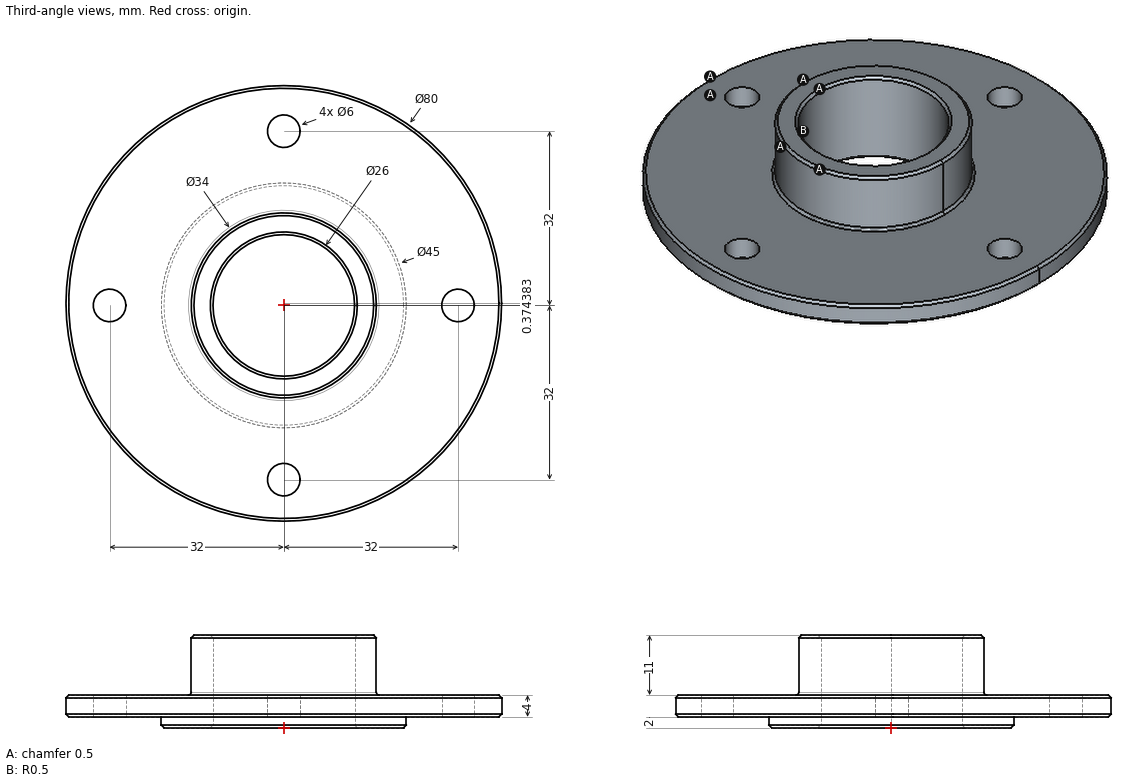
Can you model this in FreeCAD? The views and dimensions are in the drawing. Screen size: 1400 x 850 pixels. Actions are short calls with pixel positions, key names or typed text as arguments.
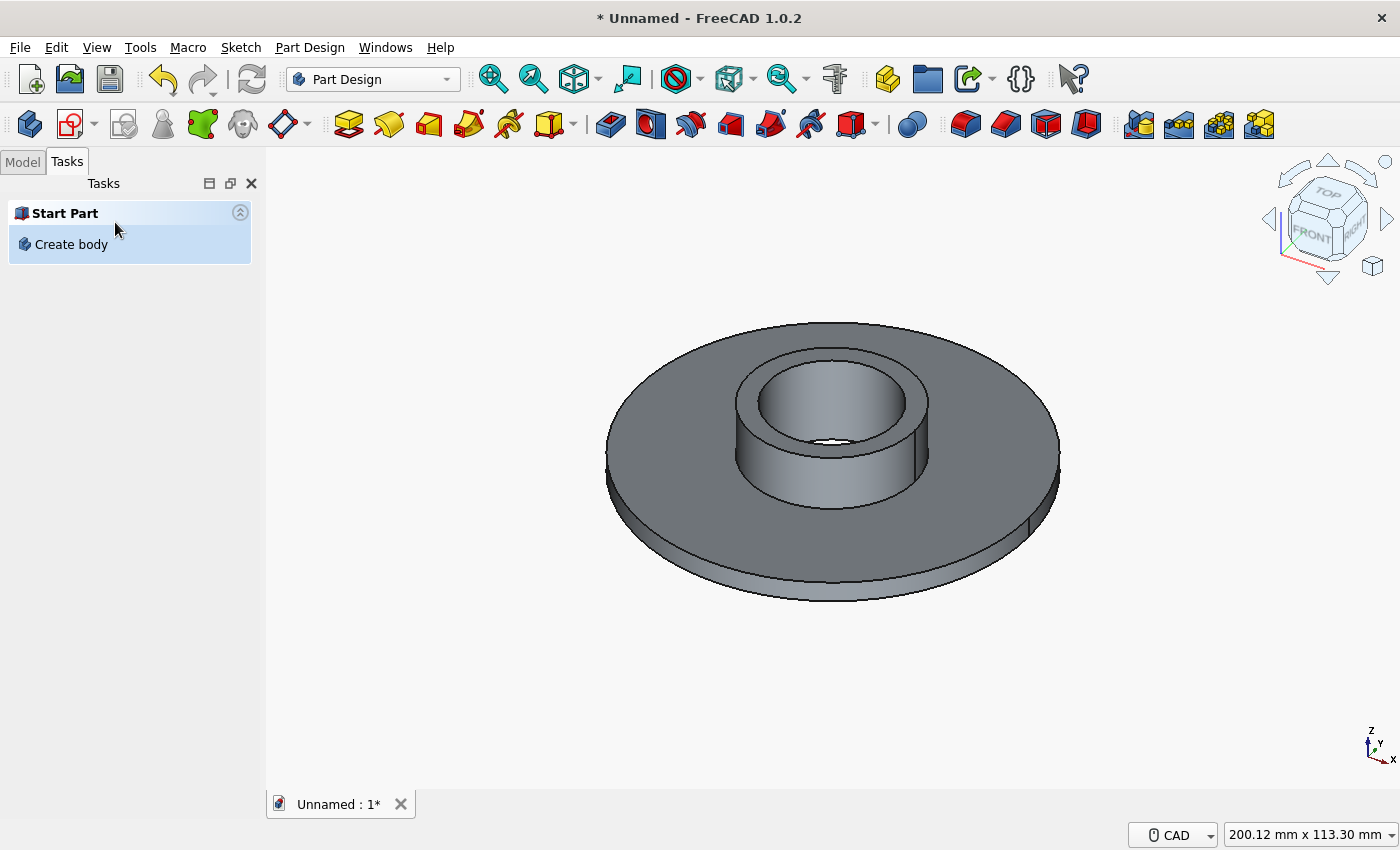
click(736, 407)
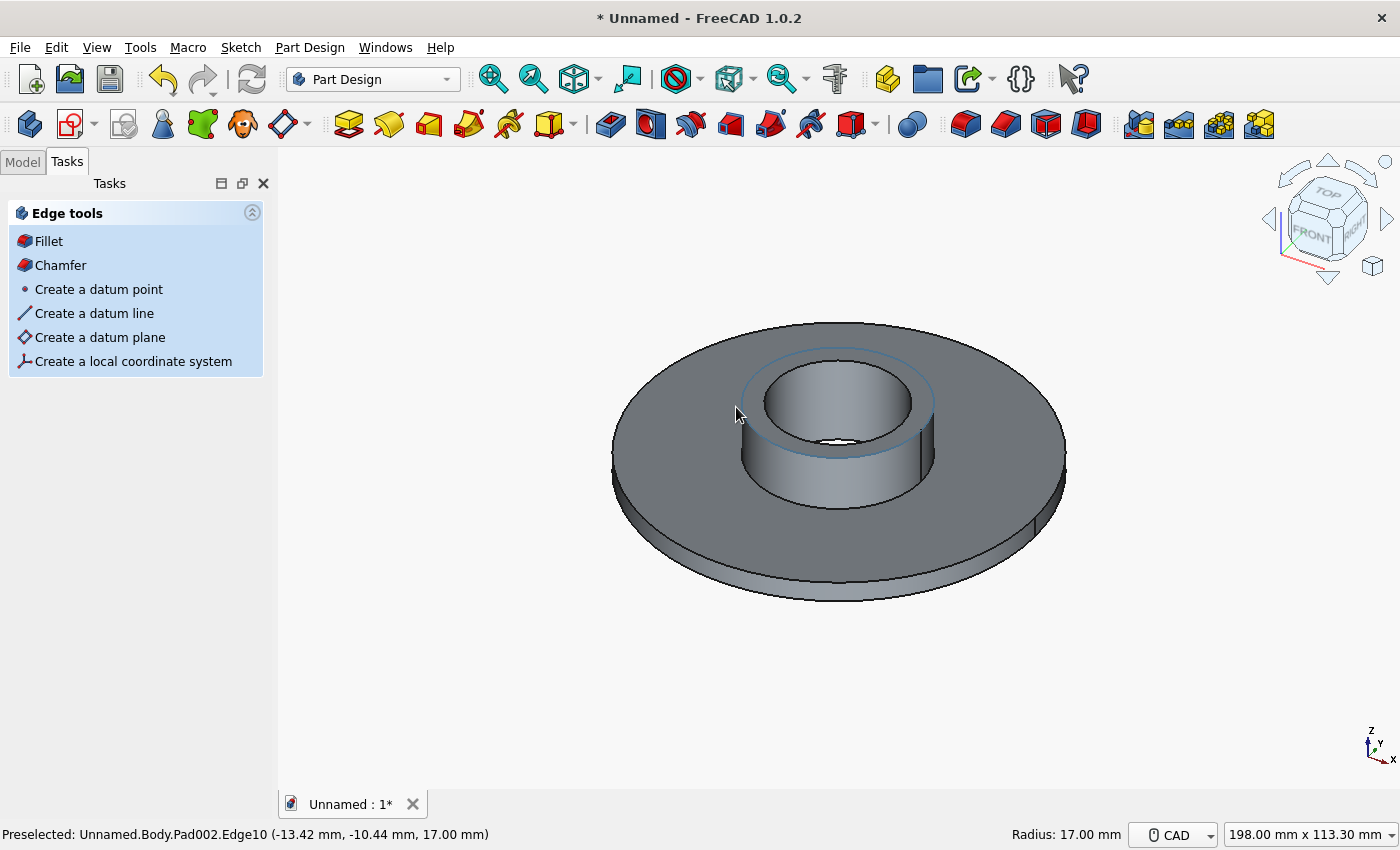
click(774, 381, ctrl)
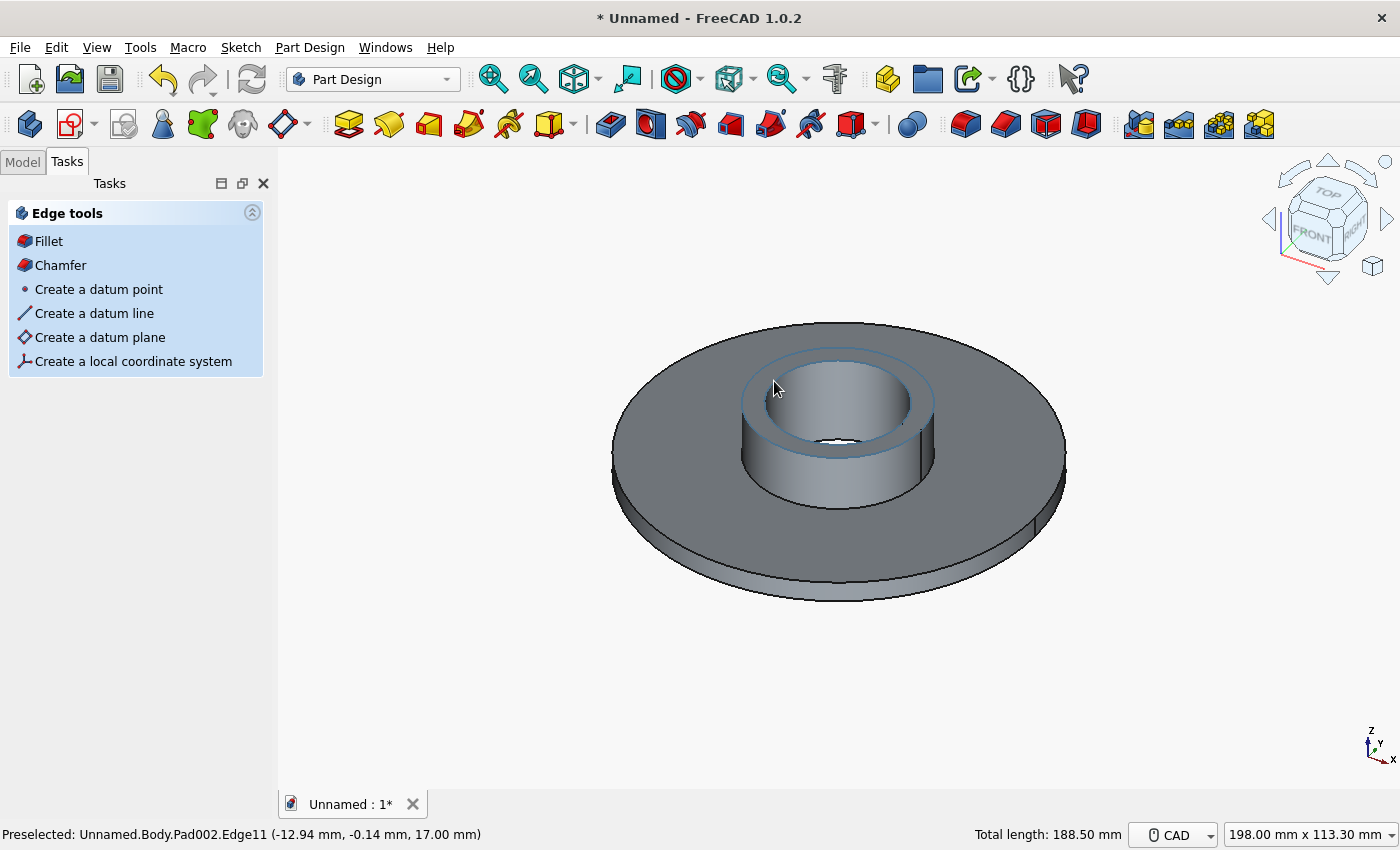
click(614, 465, ctrl)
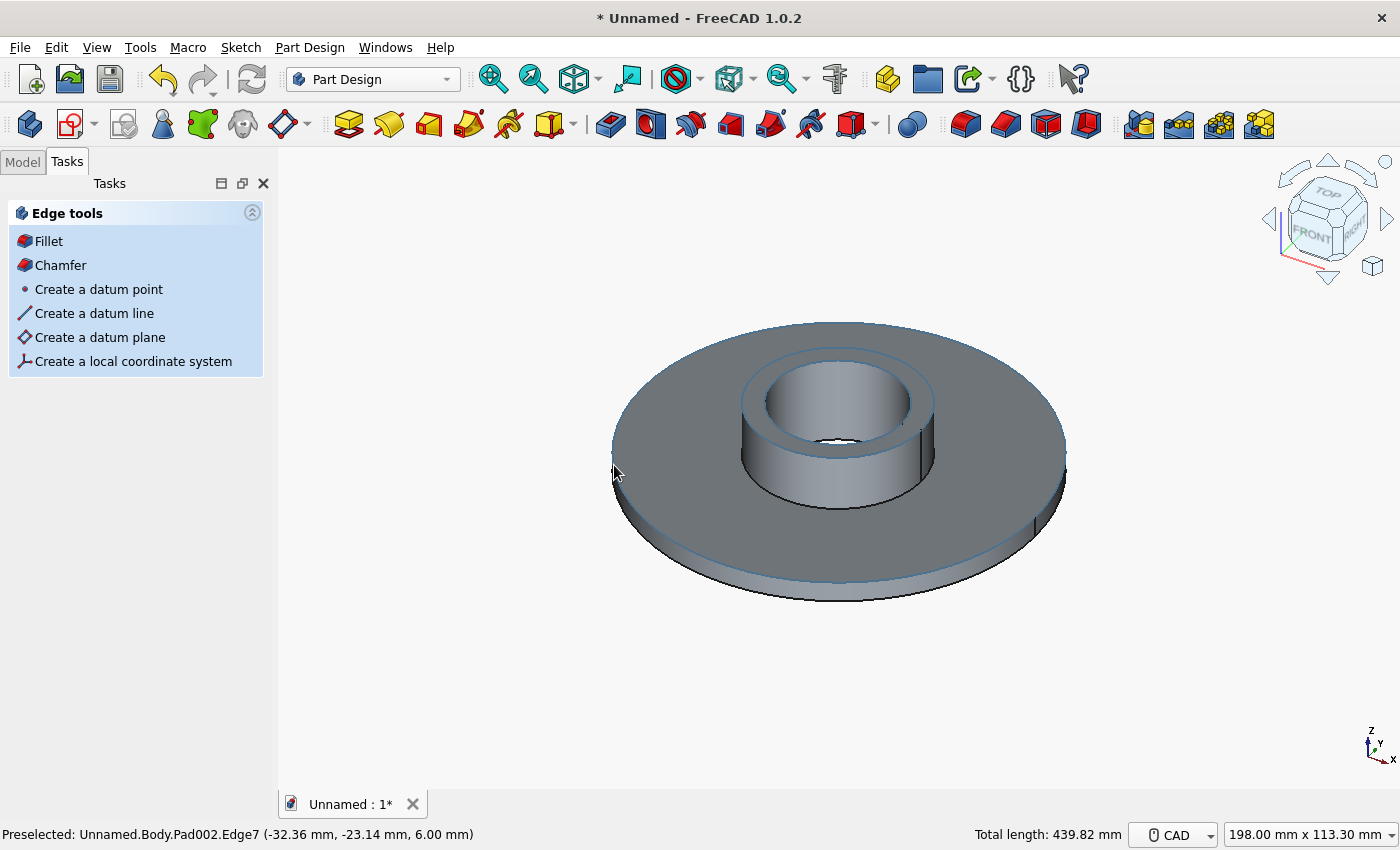
key(0)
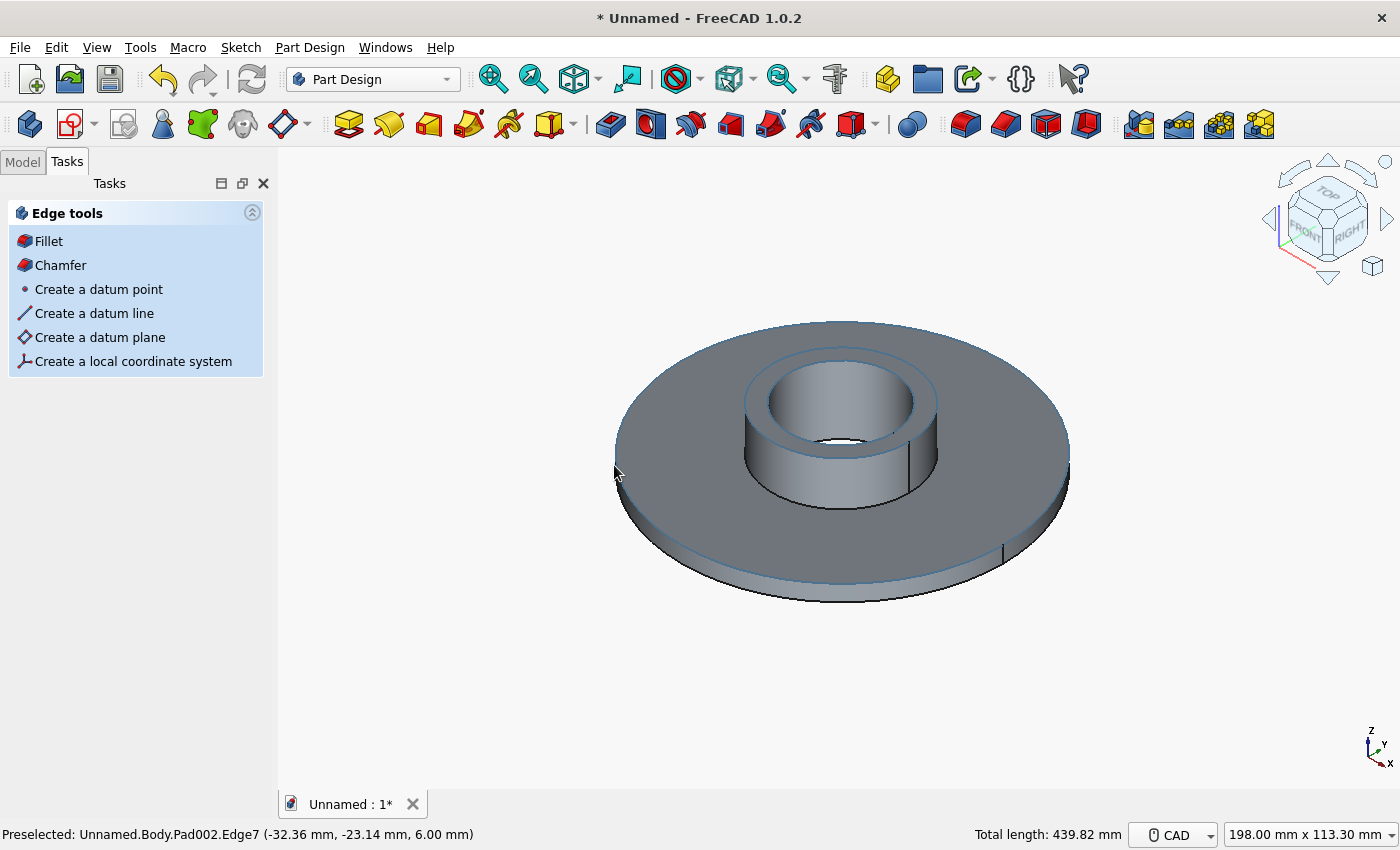
key(2)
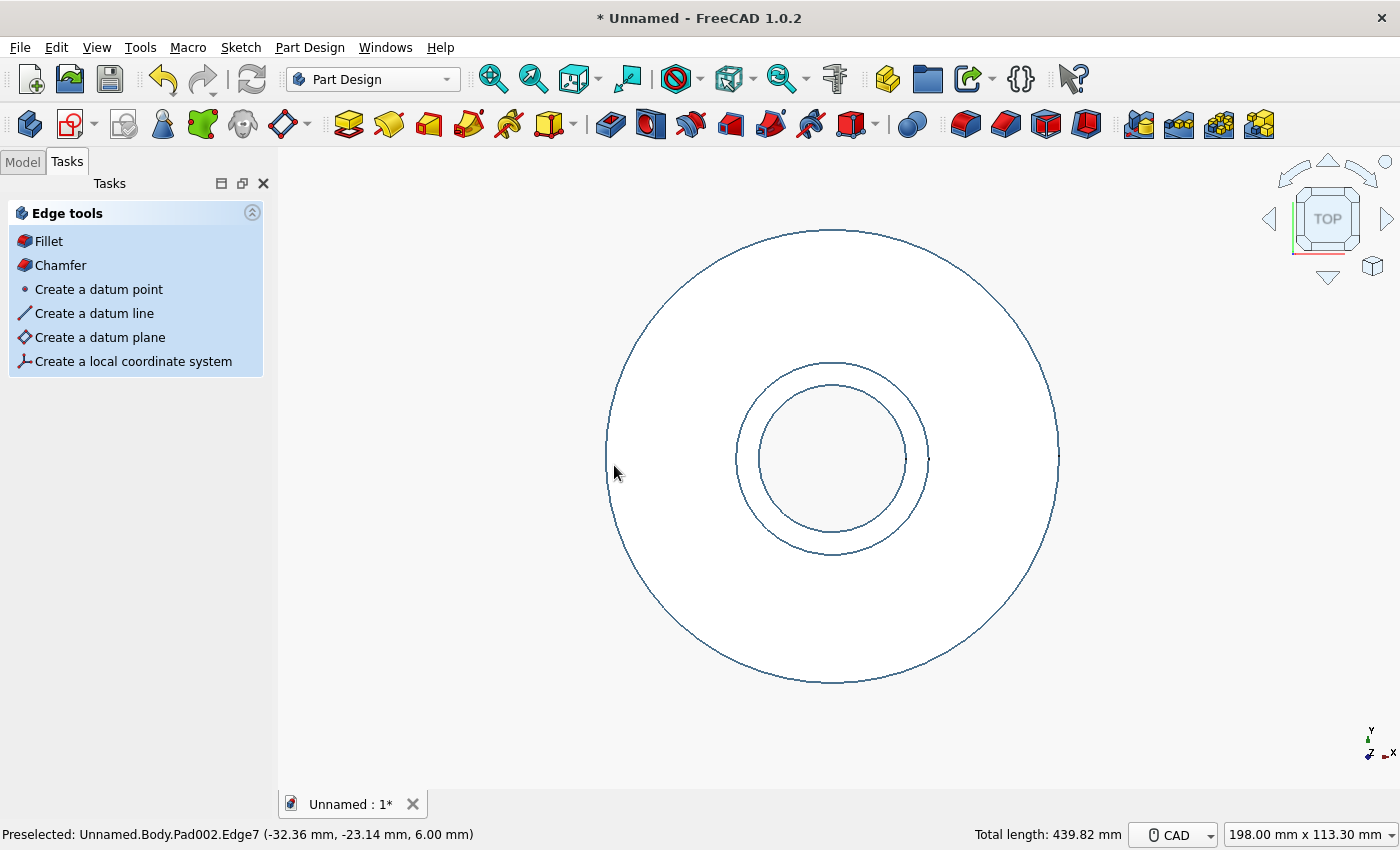
key(1)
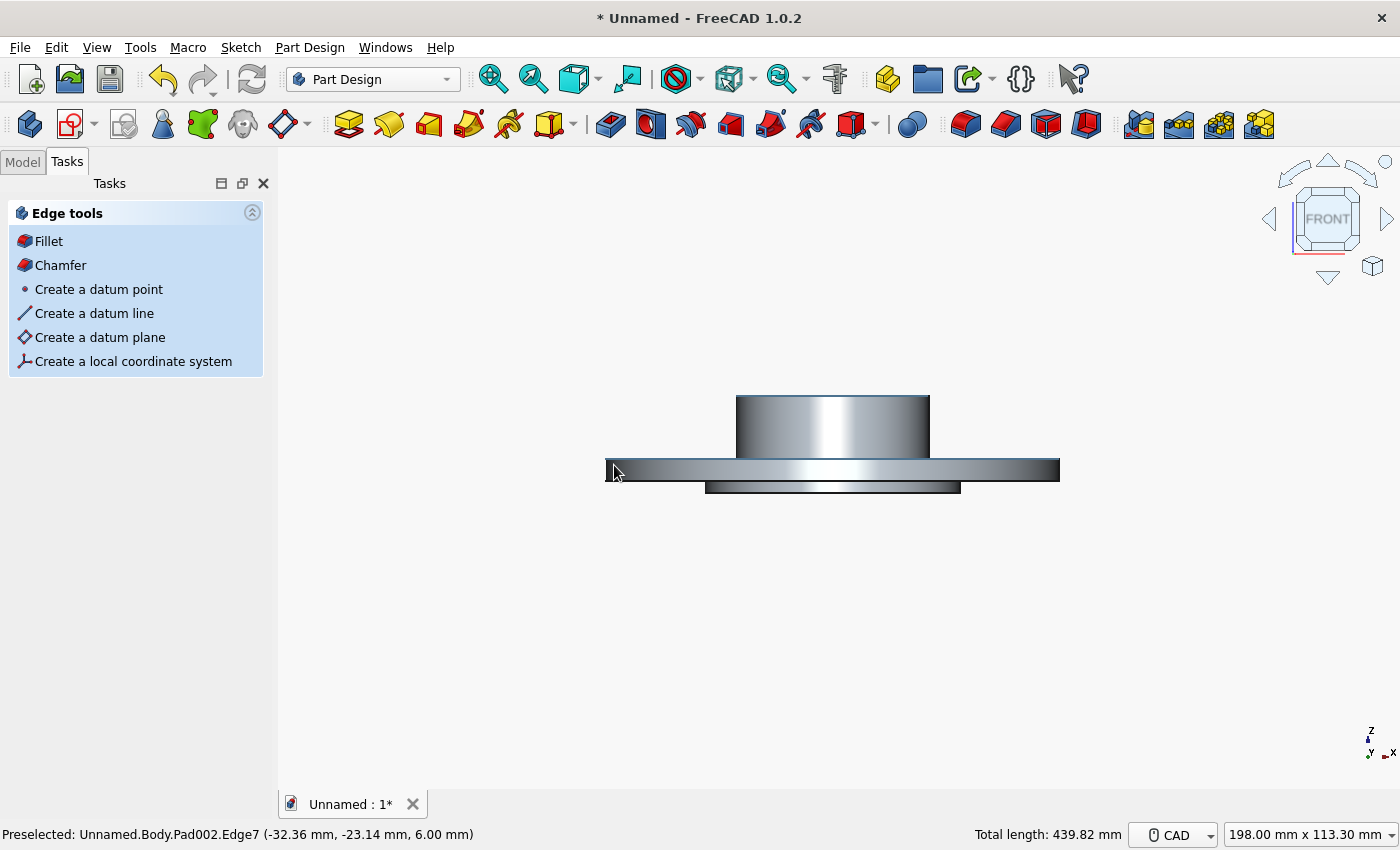
click(494, 80)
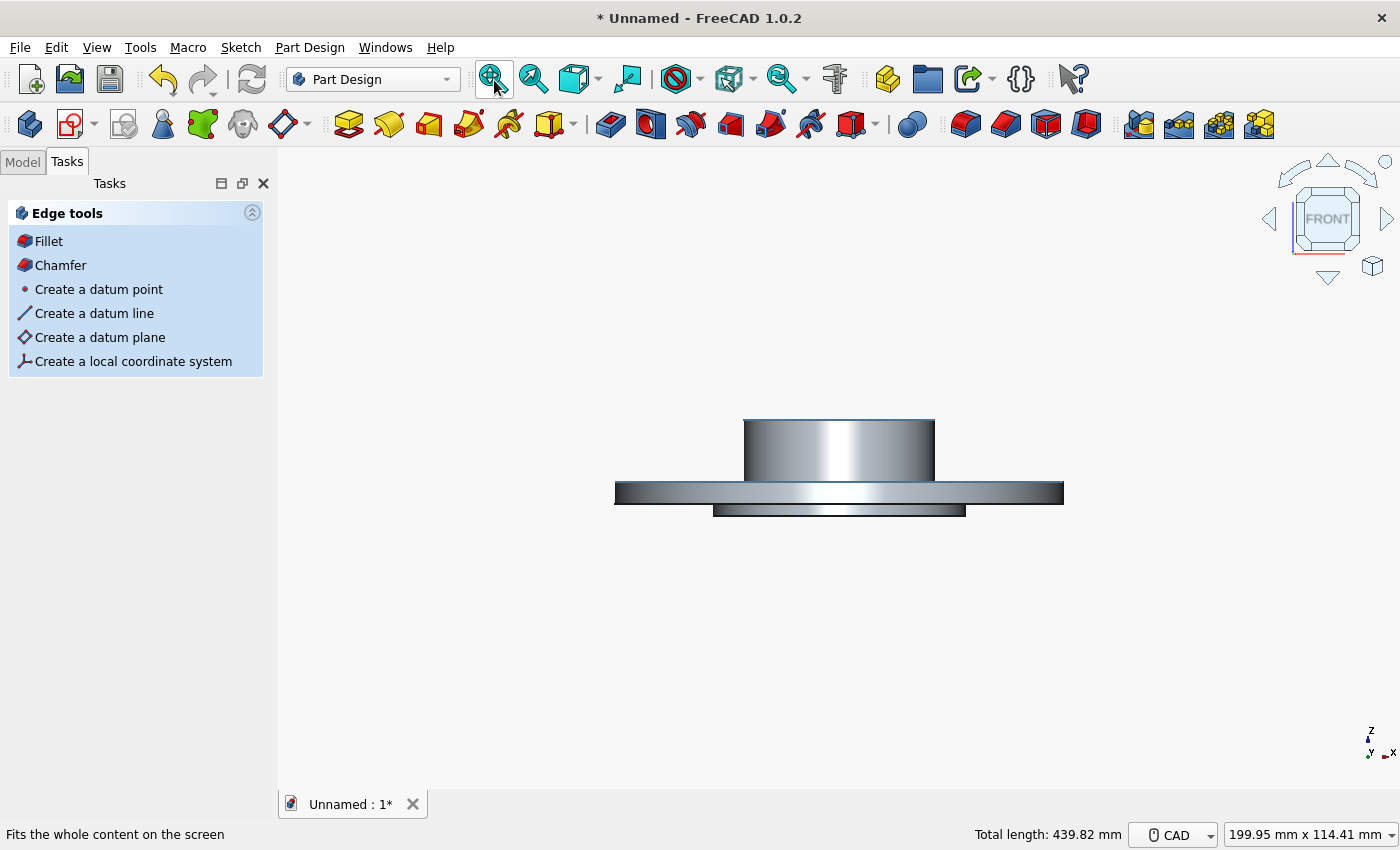
click(657, 503, ctrl)